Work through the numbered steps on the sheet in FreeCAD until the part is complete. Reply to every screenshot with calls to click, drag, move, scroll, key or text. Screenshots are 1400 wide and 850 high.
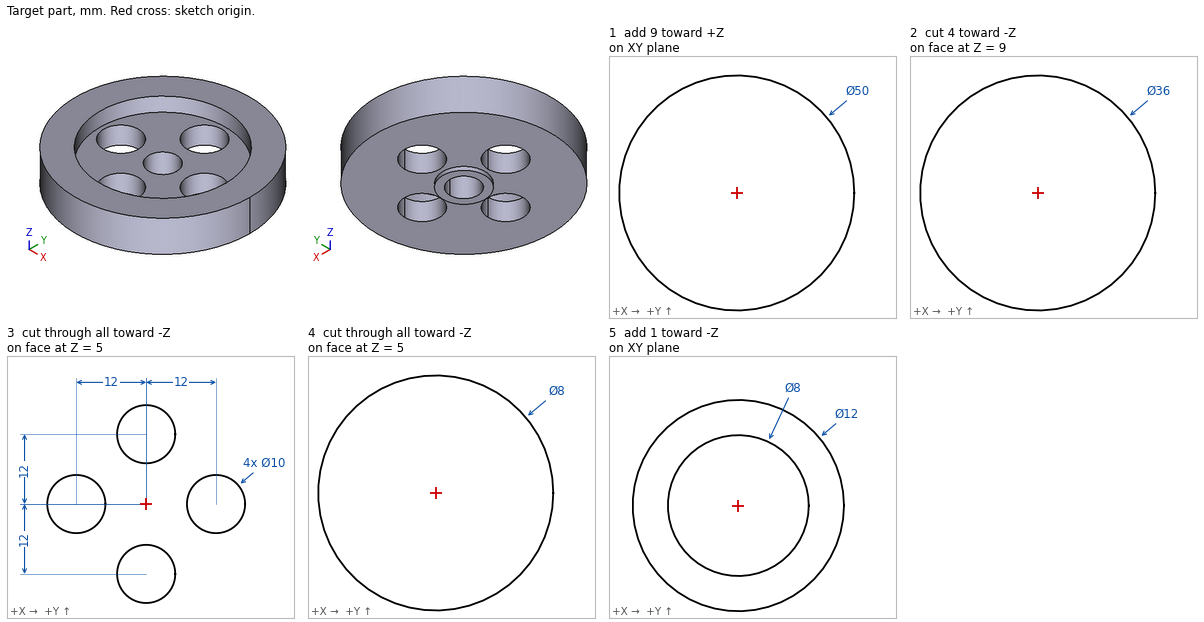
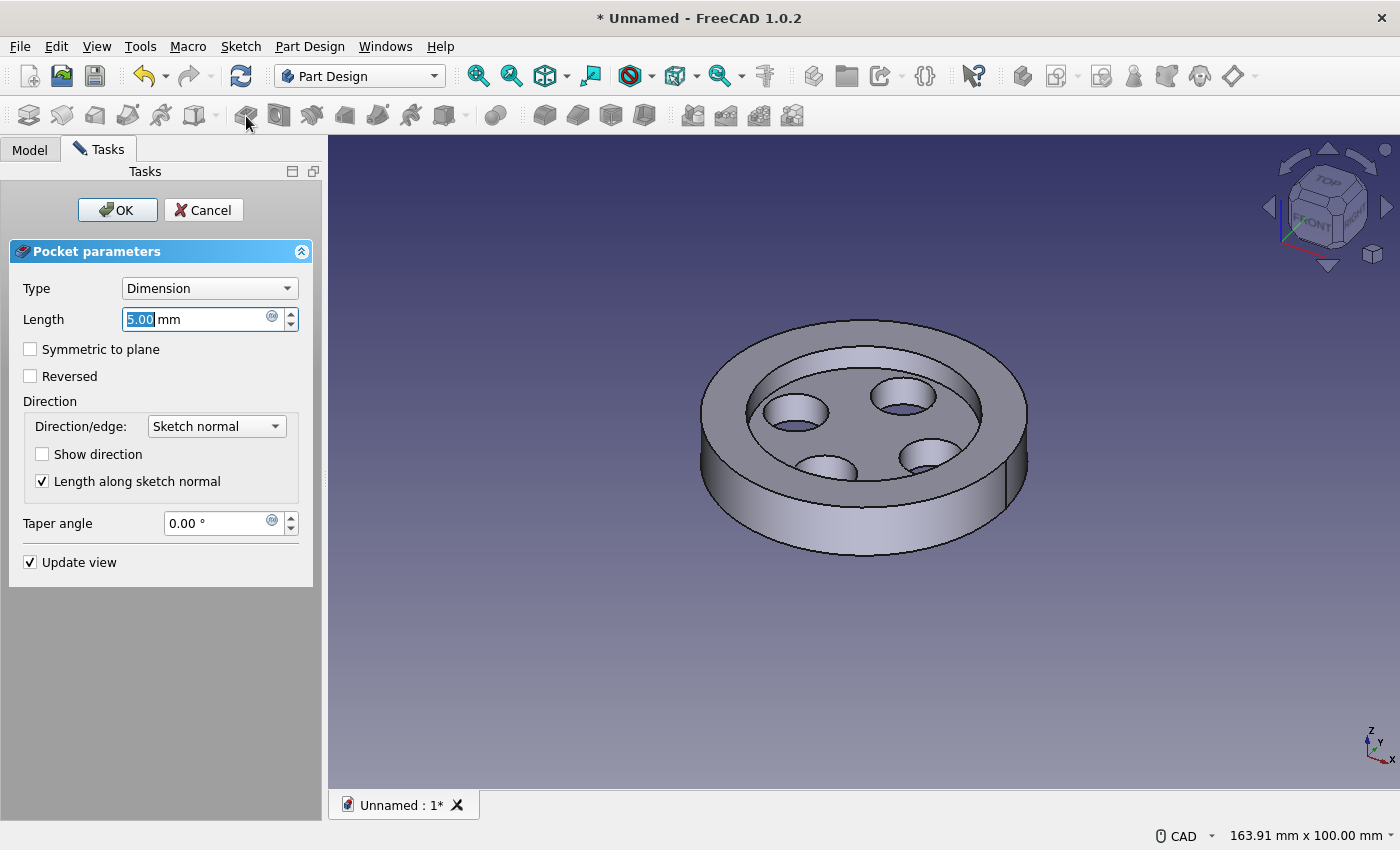
click(210, 288)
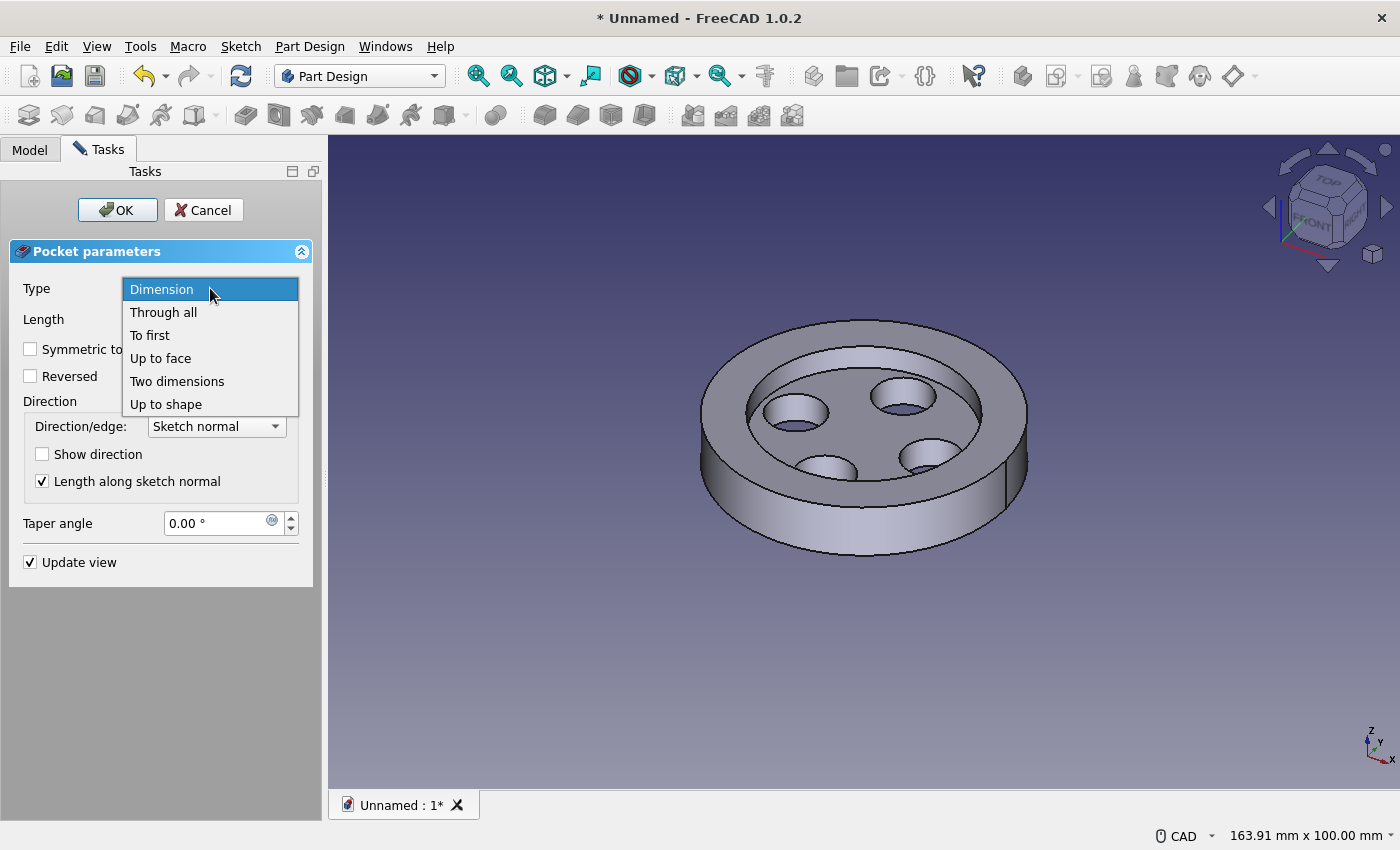
click(208, 312)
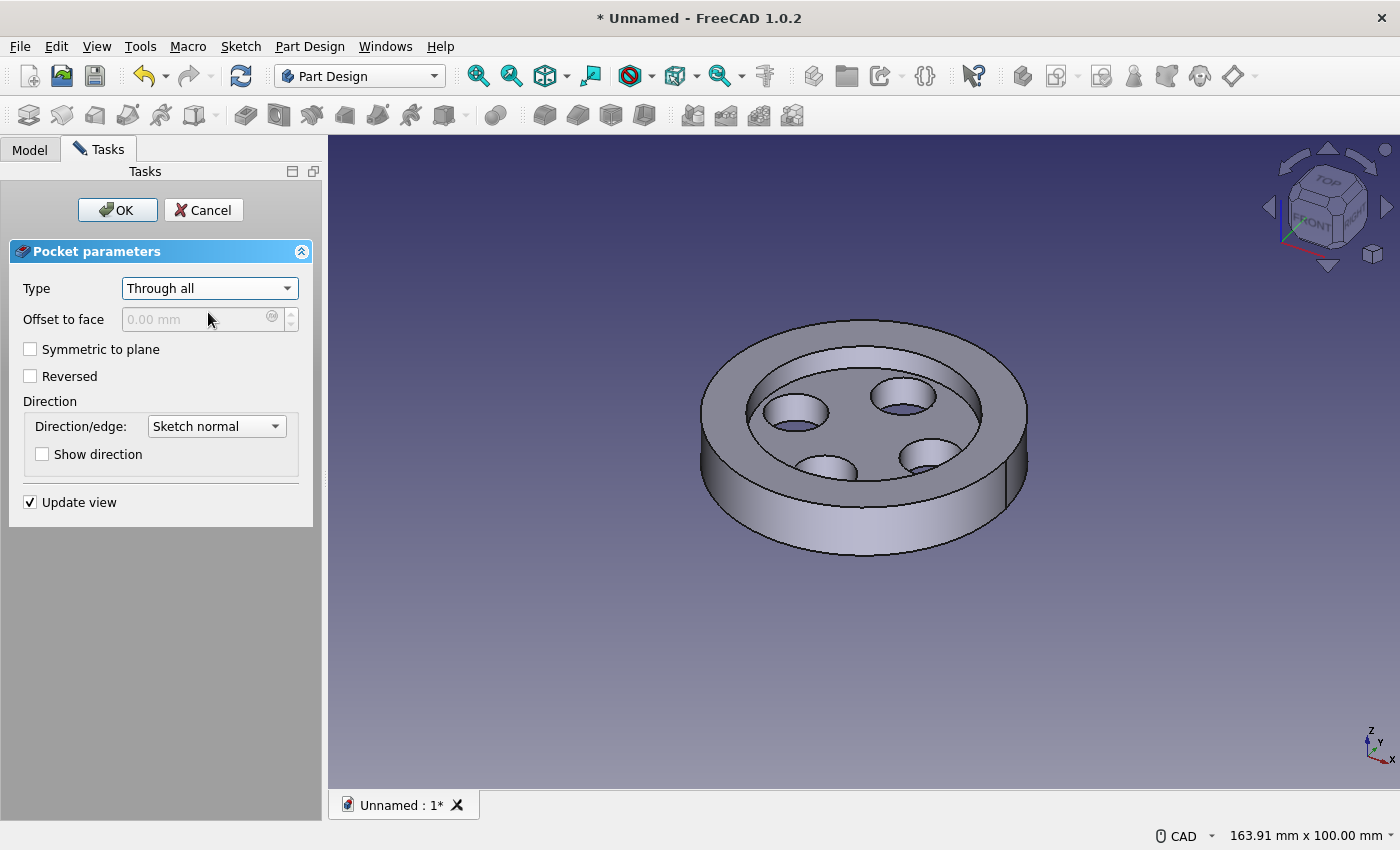
click(118, 210)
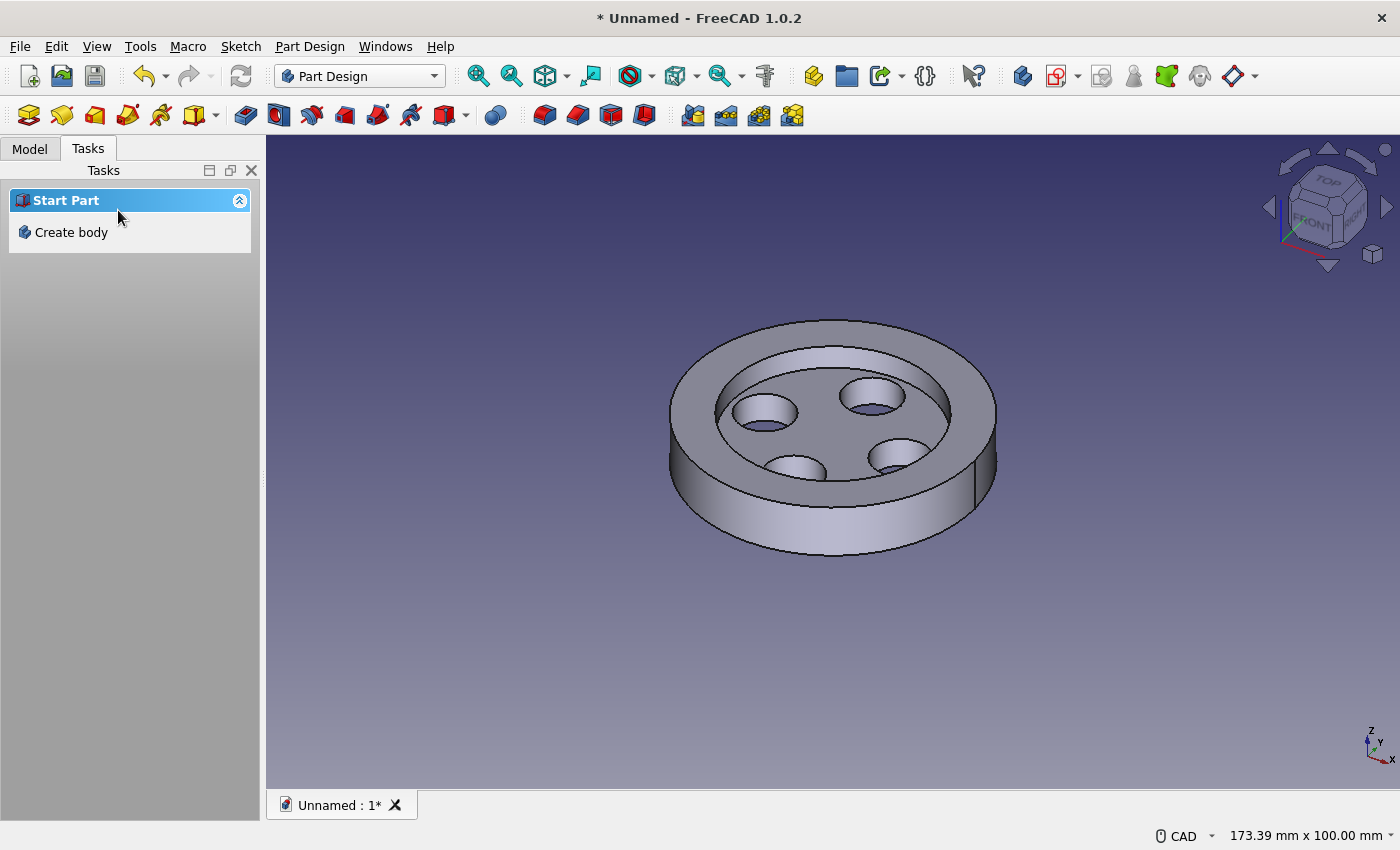
click(833, 434)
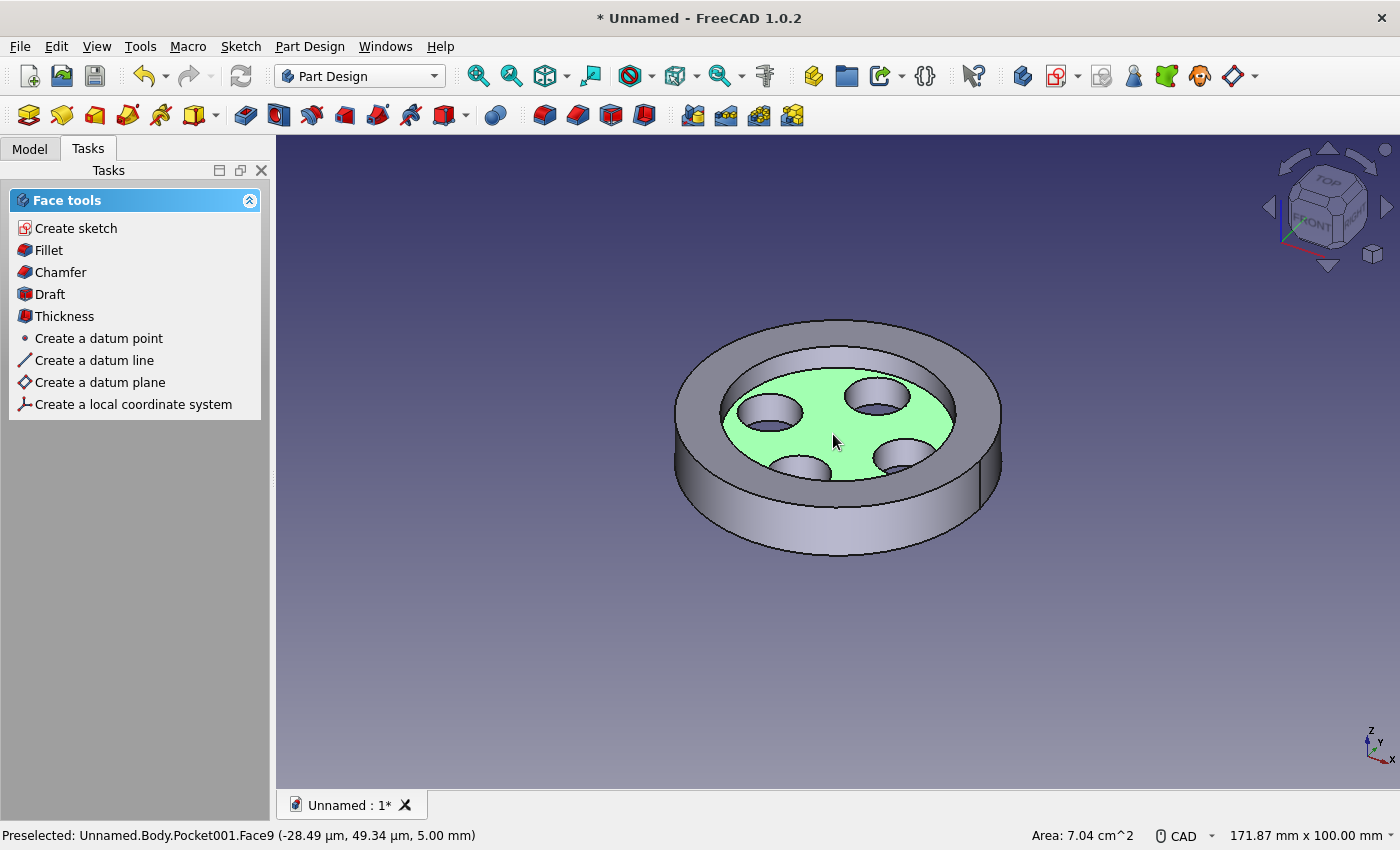
click(1056, 76)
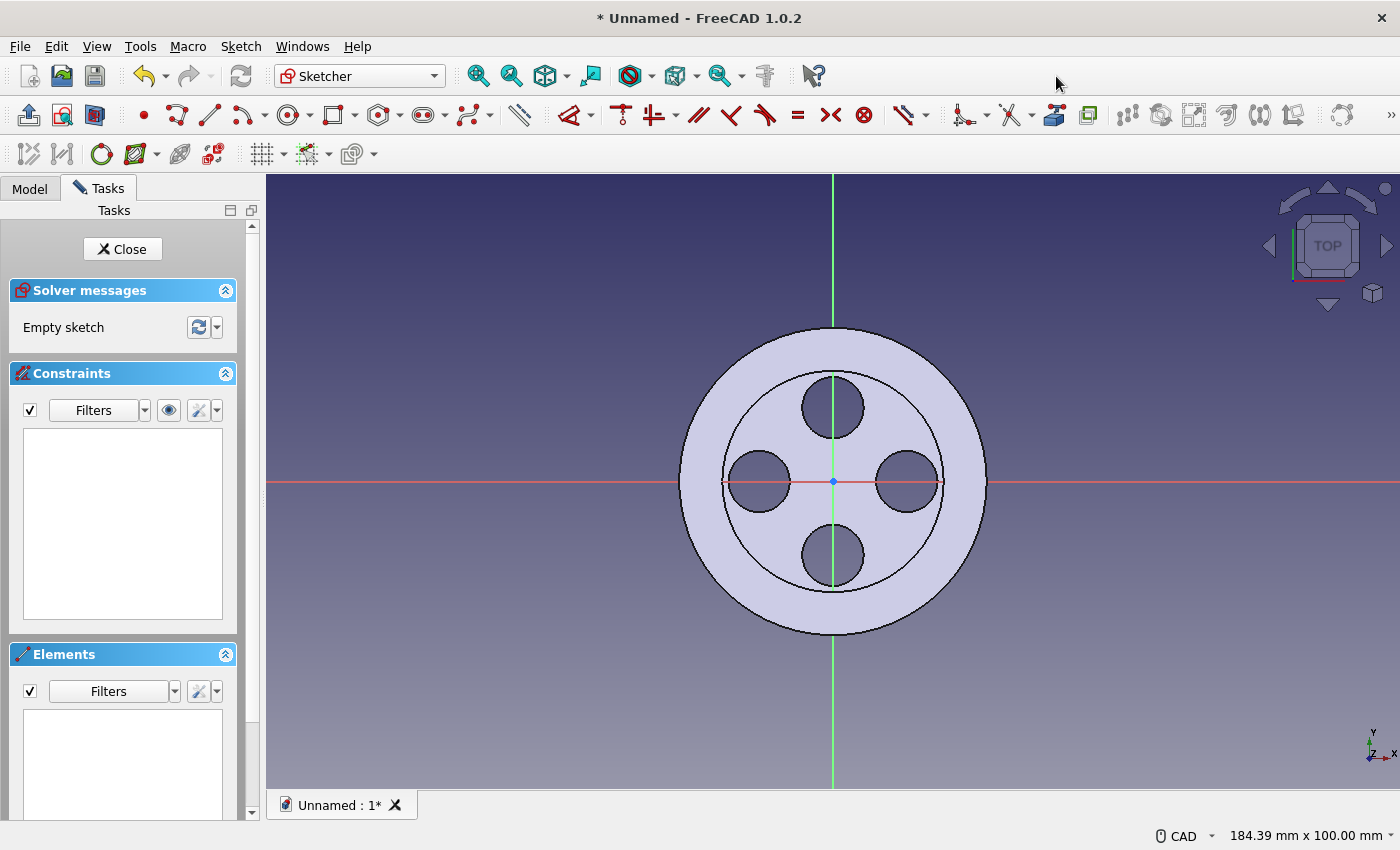
click(95, 116)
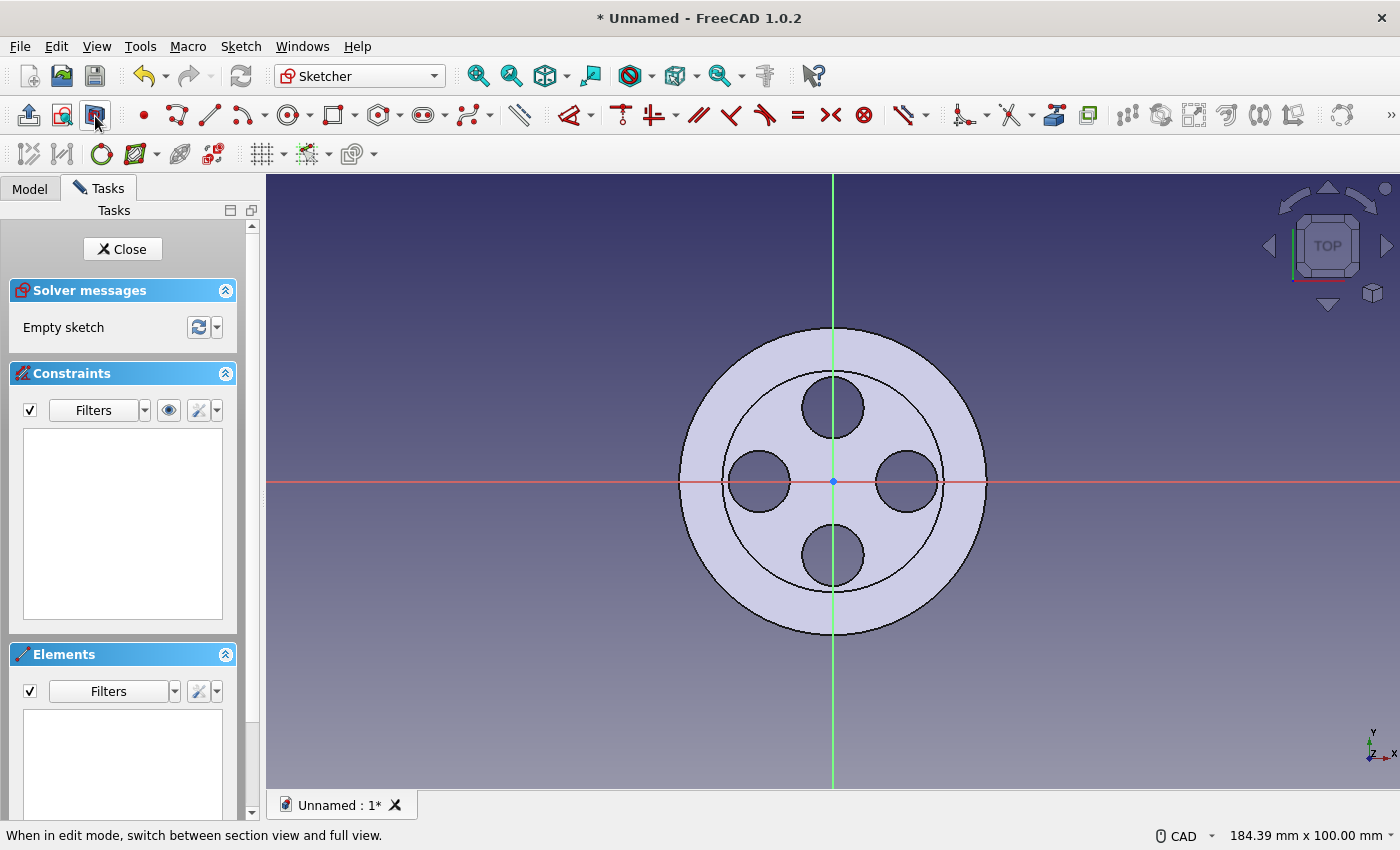
scroll(844, 482, up, 10)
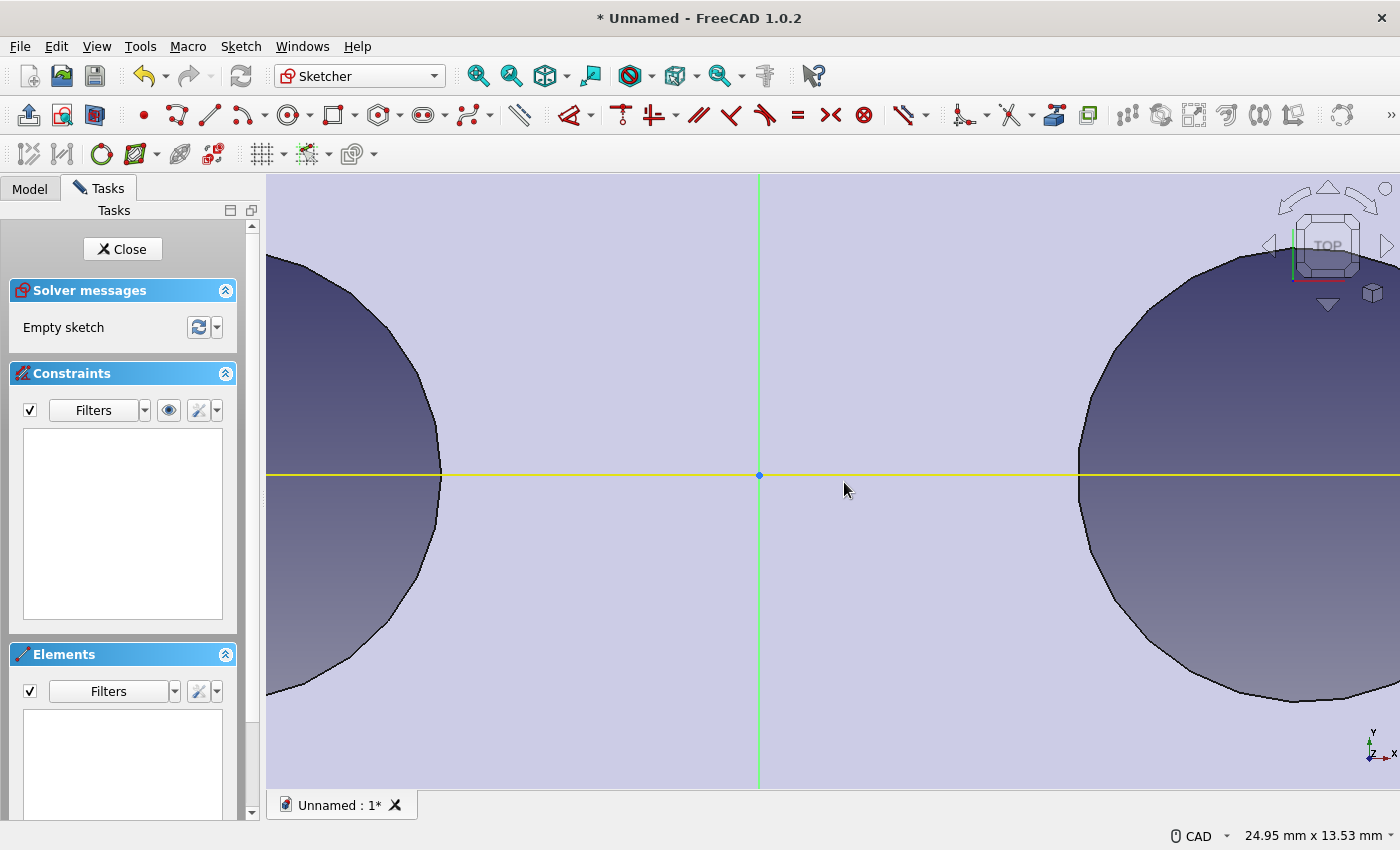
click(288, 116)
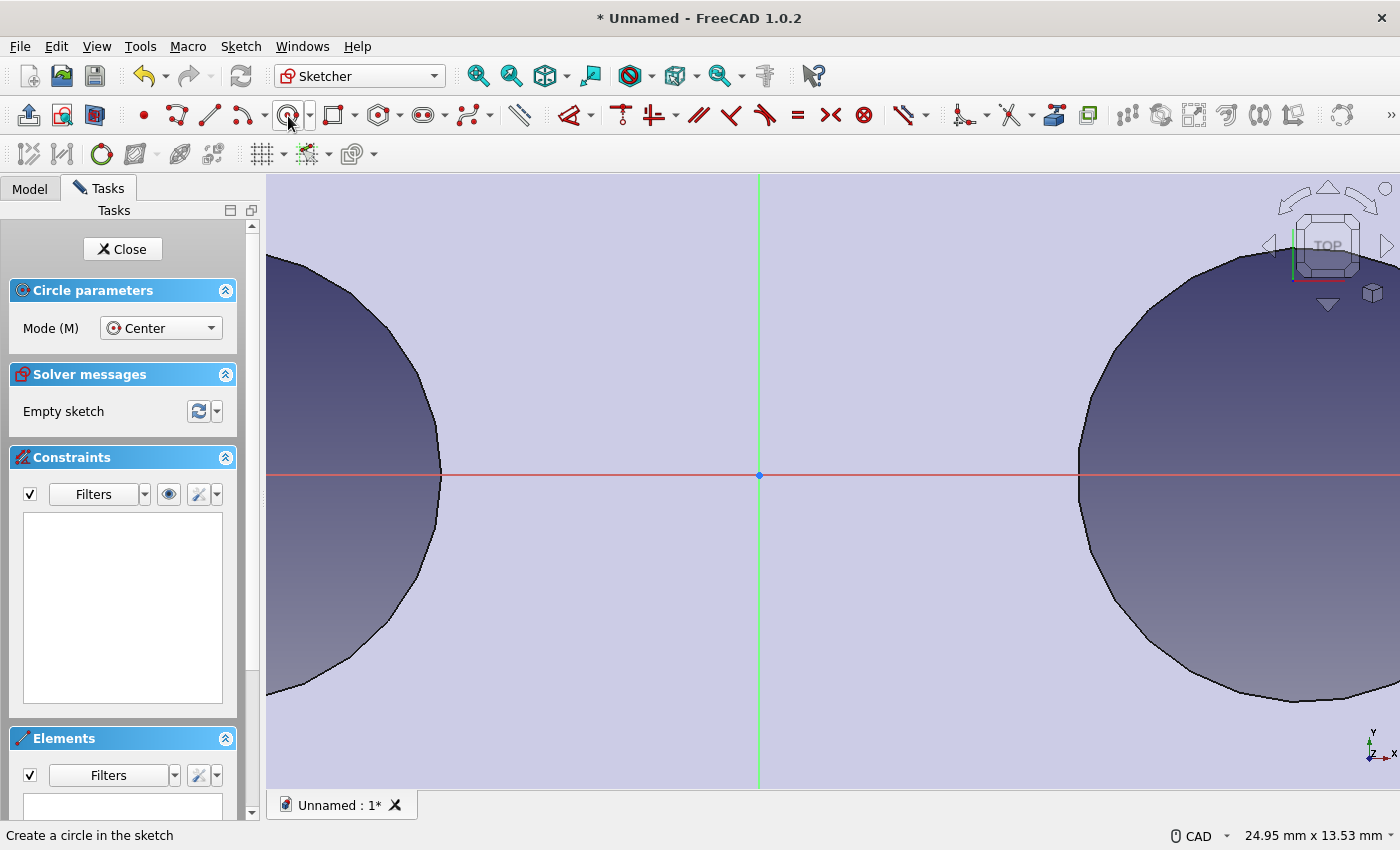
click(759, 475)
move(888, 347)